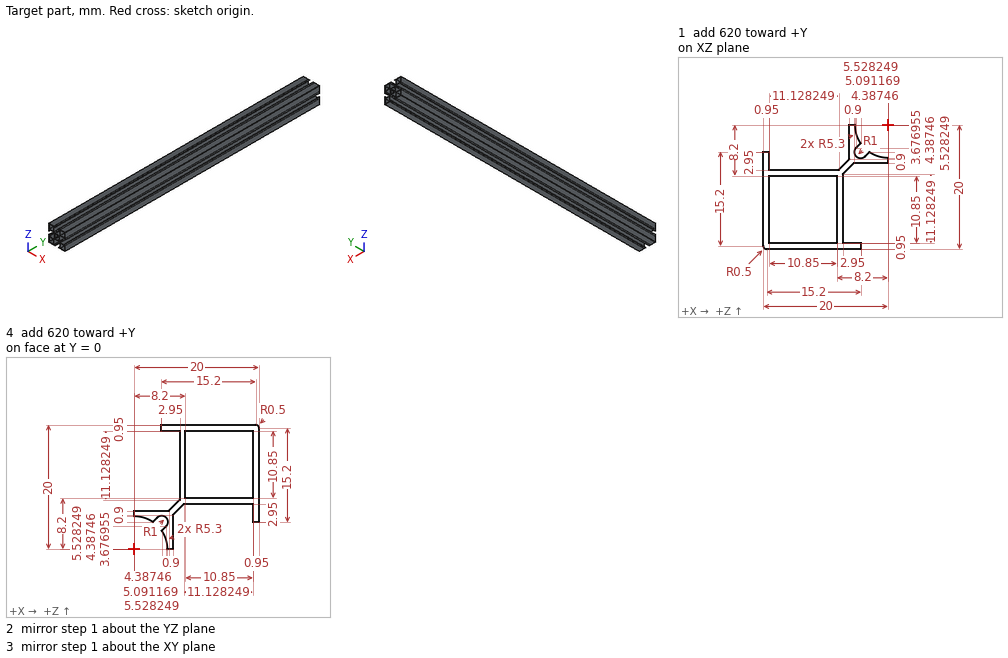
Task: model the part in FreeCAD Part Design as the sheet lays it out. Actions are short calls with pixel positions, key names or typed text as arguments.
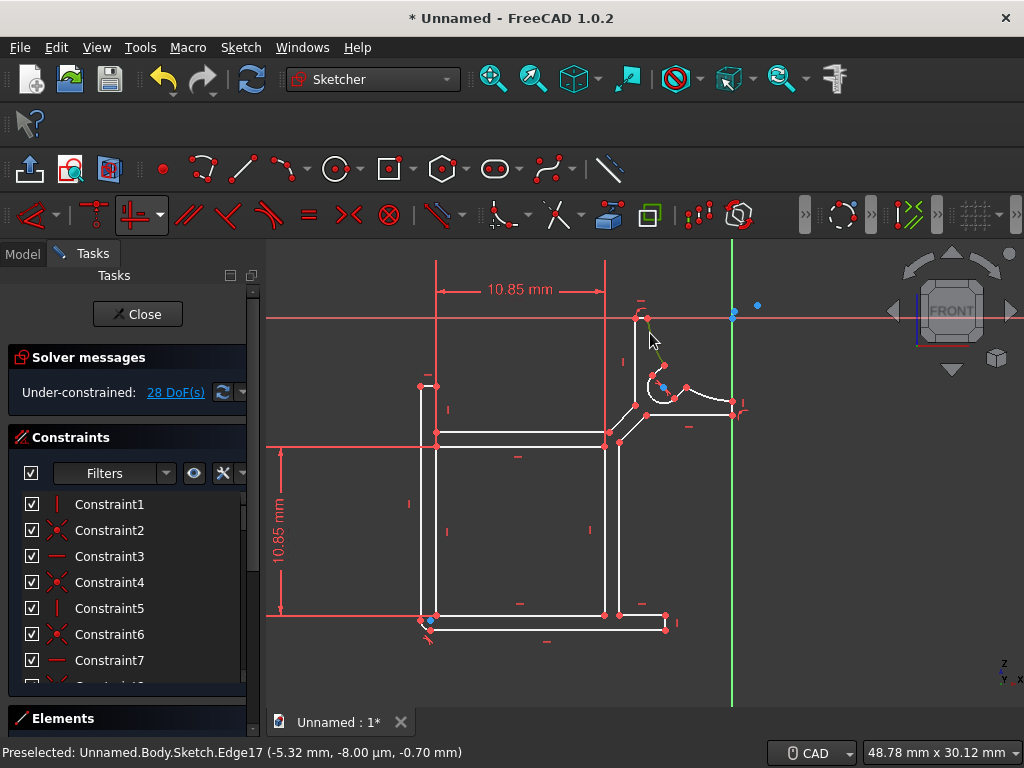
click(699, 394)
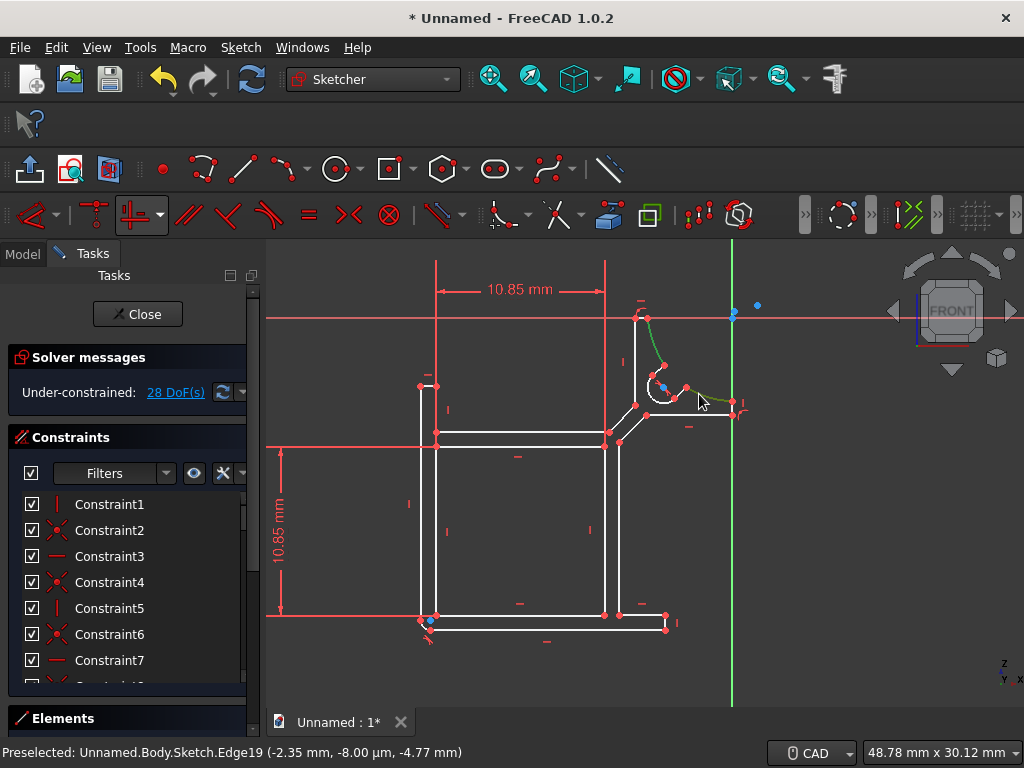
click(94, 216)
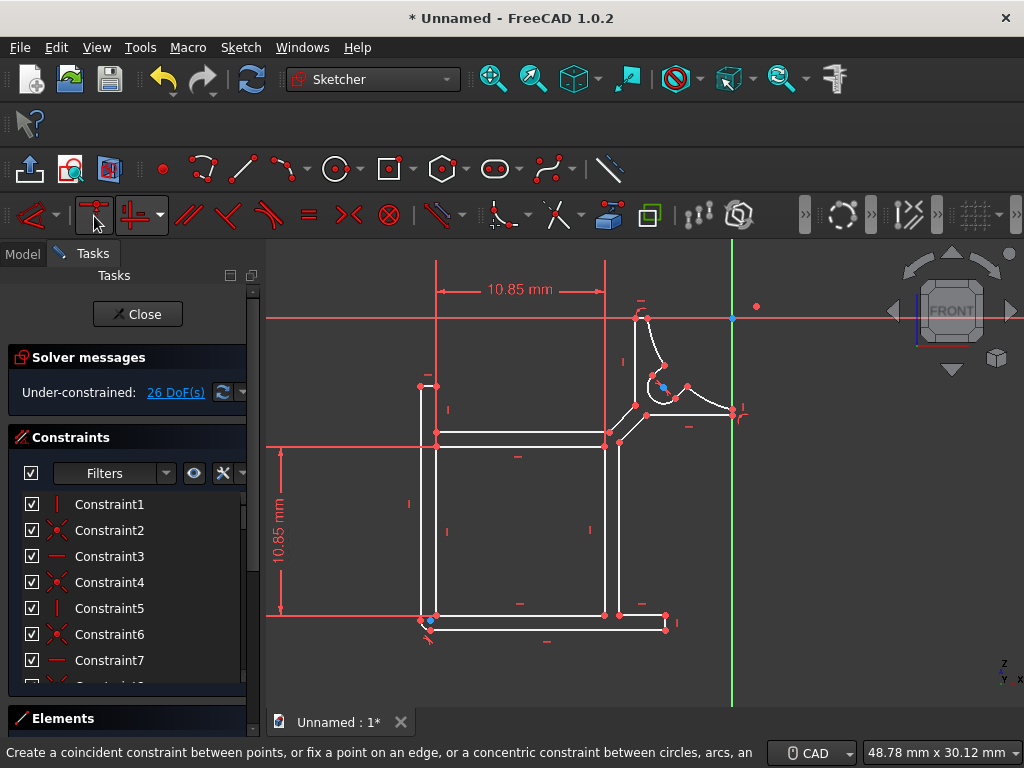
scroll(744, 312, up, 7)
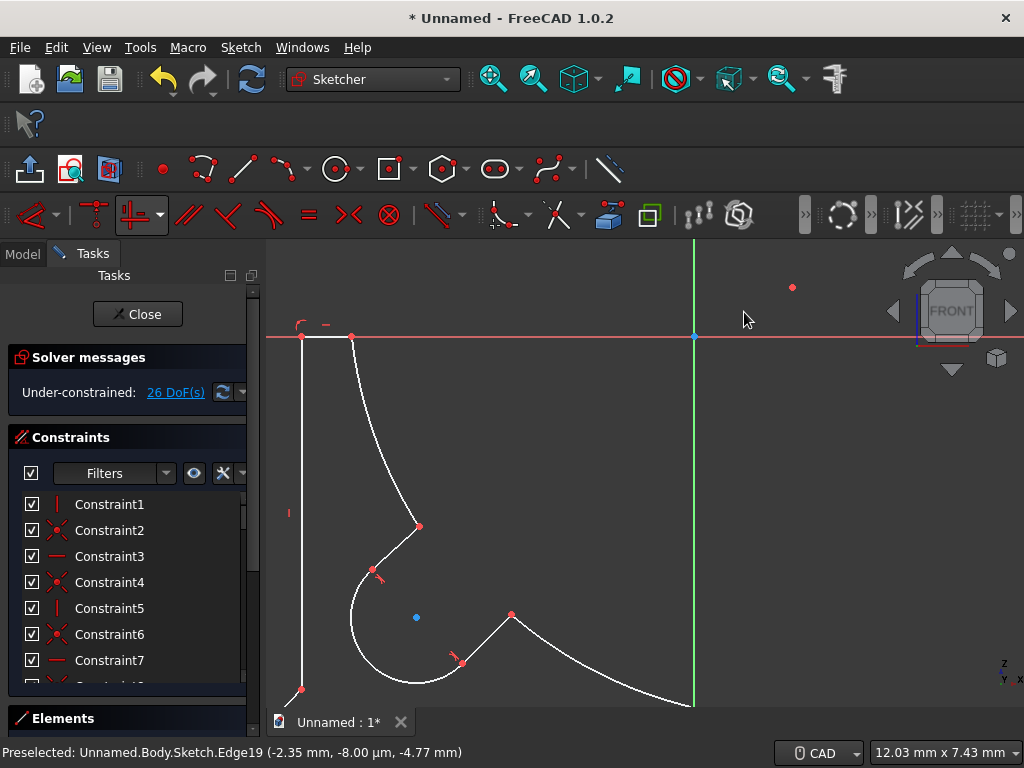
drag(684, 278, 803, 347)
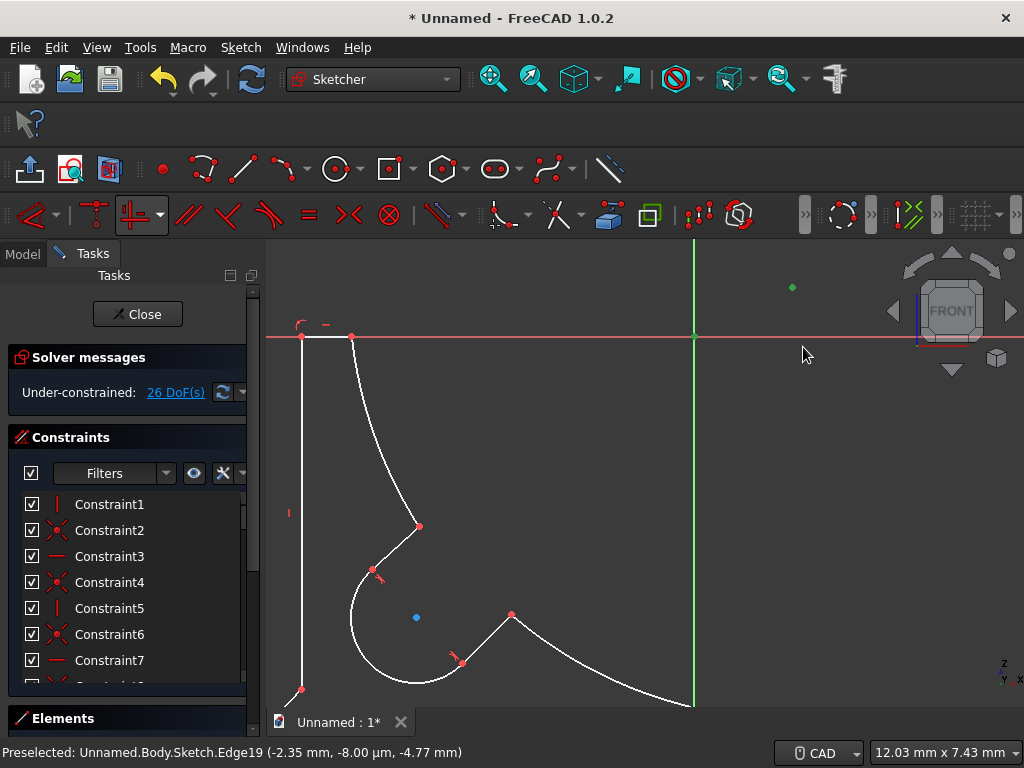
click(94, 216)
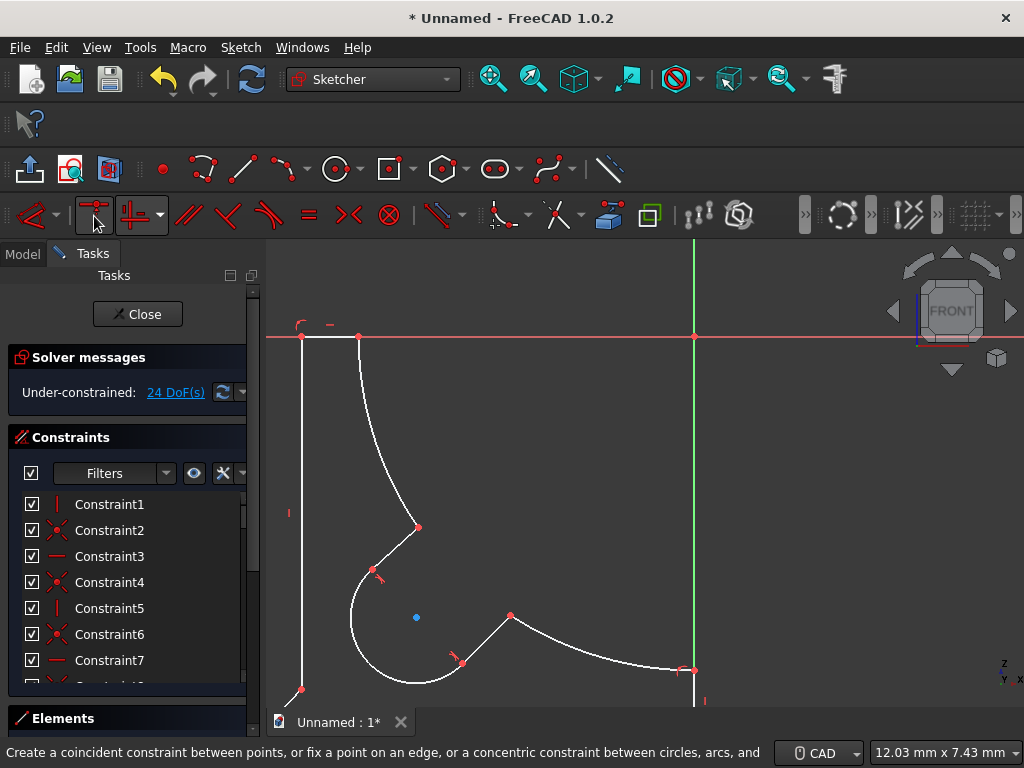
scroll(744, 311, down, 7)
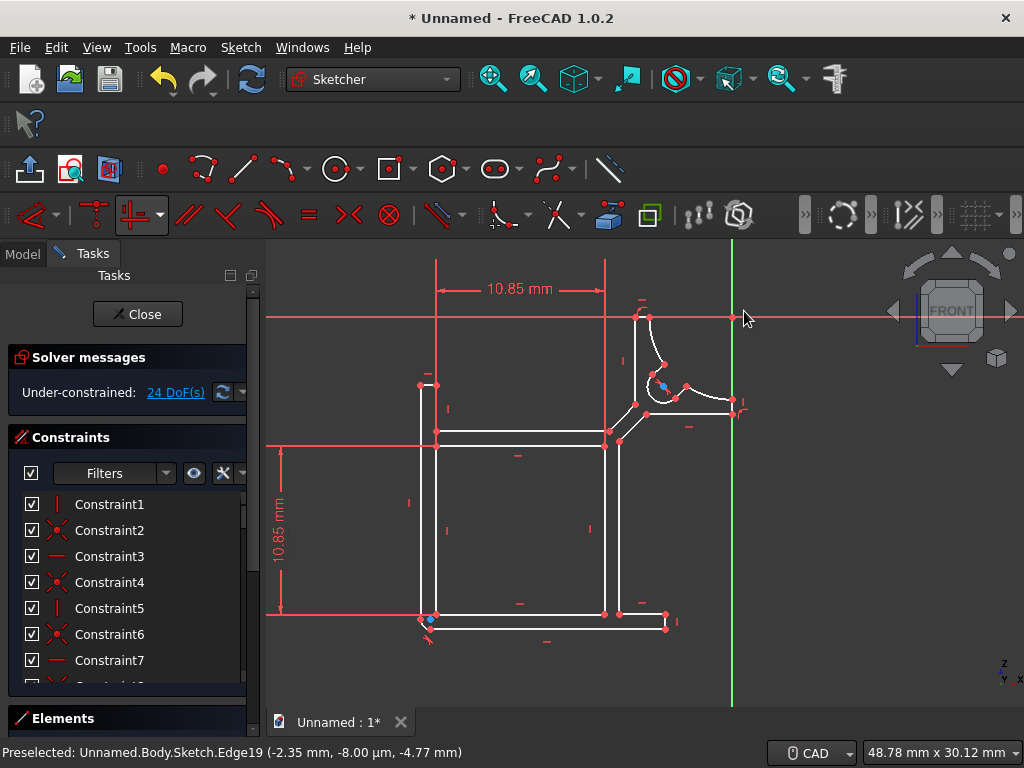
click(651, 332)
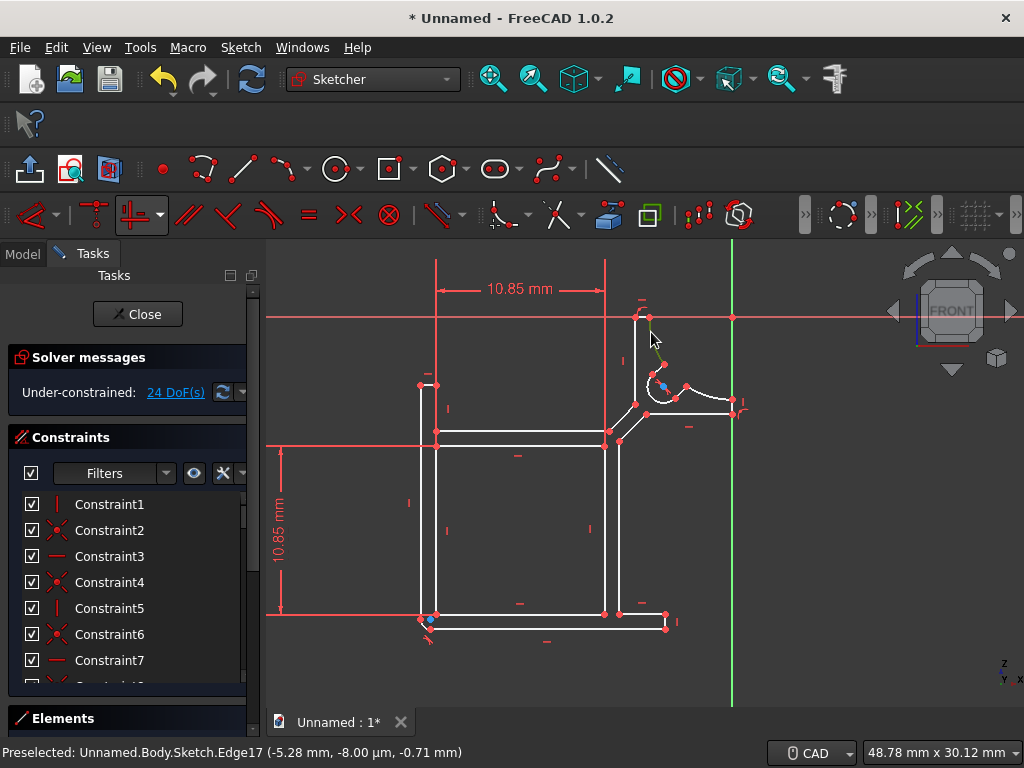
click(700, 393)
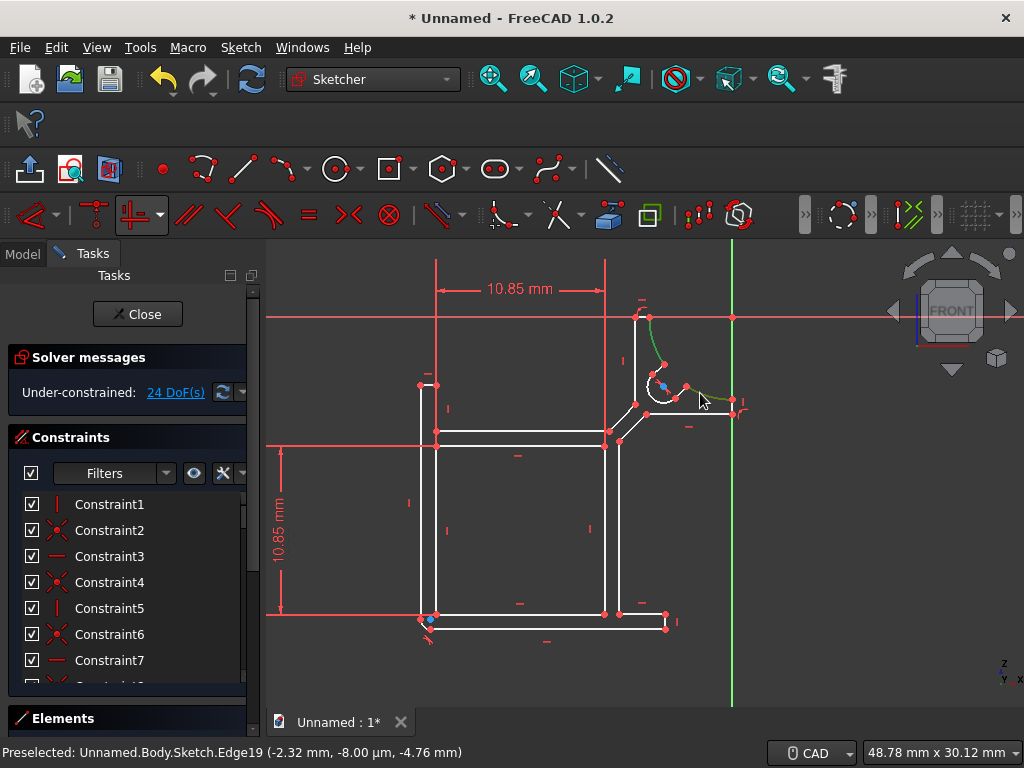
click(310, 216)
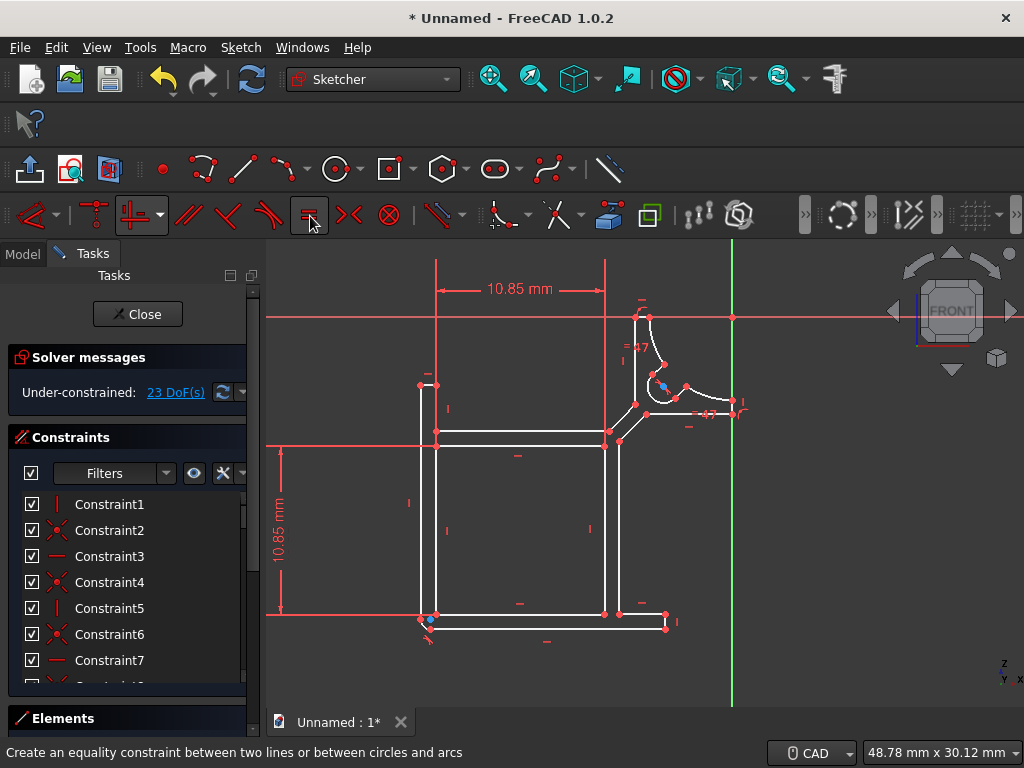
click(651, 332)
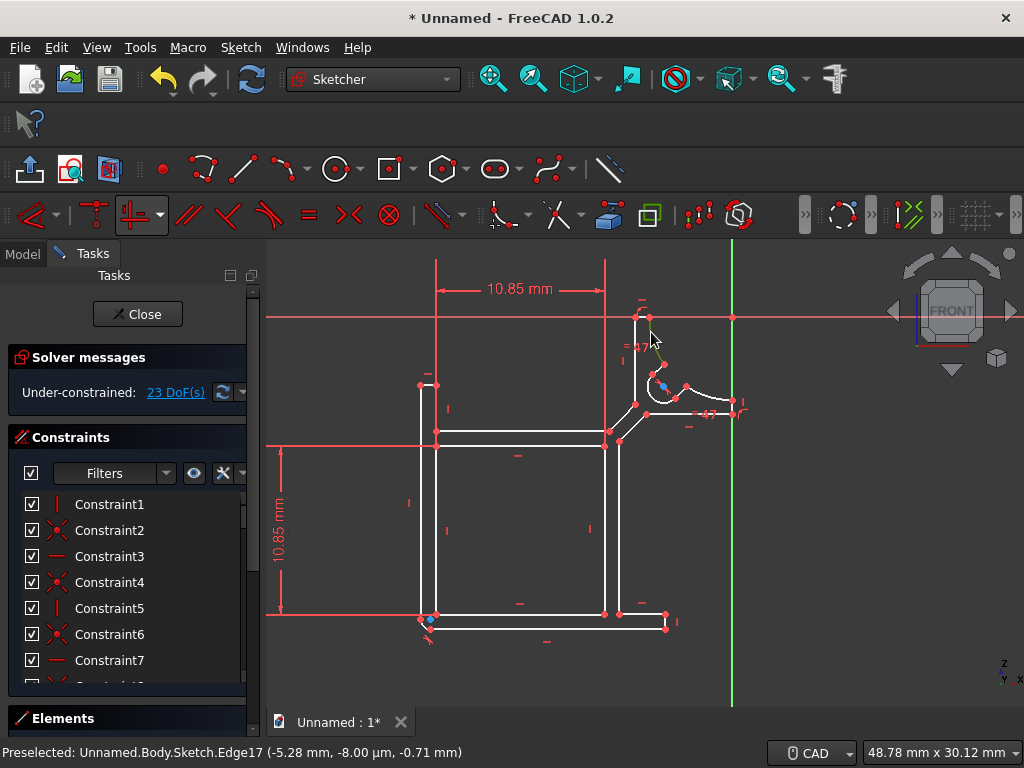
key(k)
key(r)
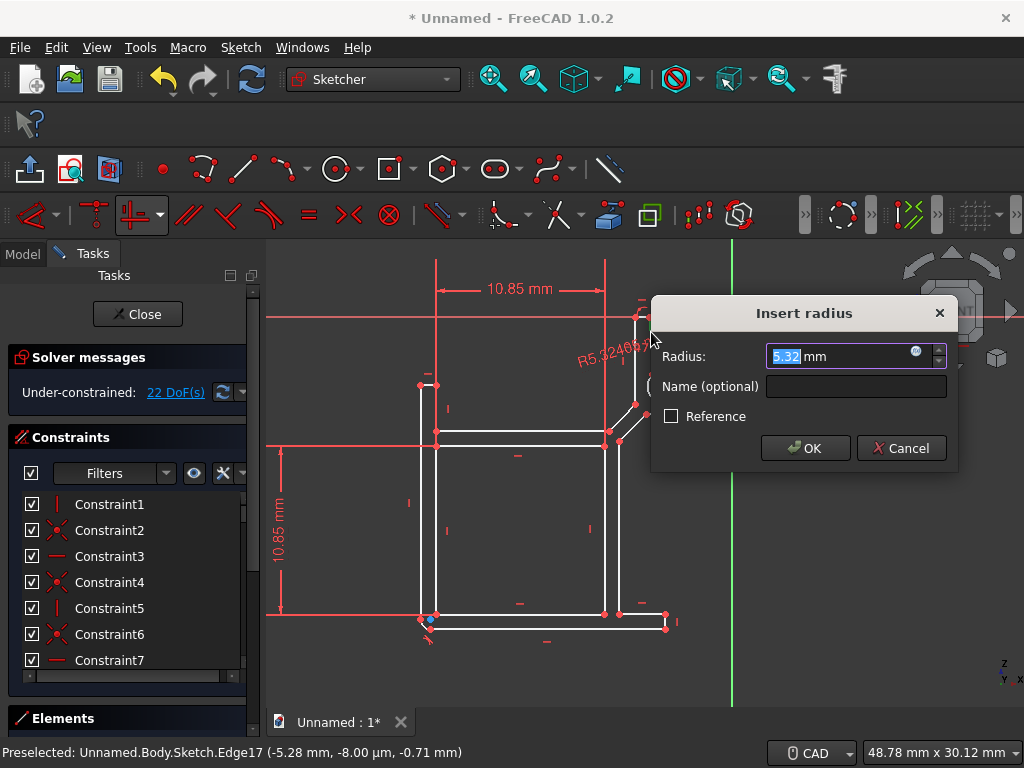
text(5.3)
key(Return)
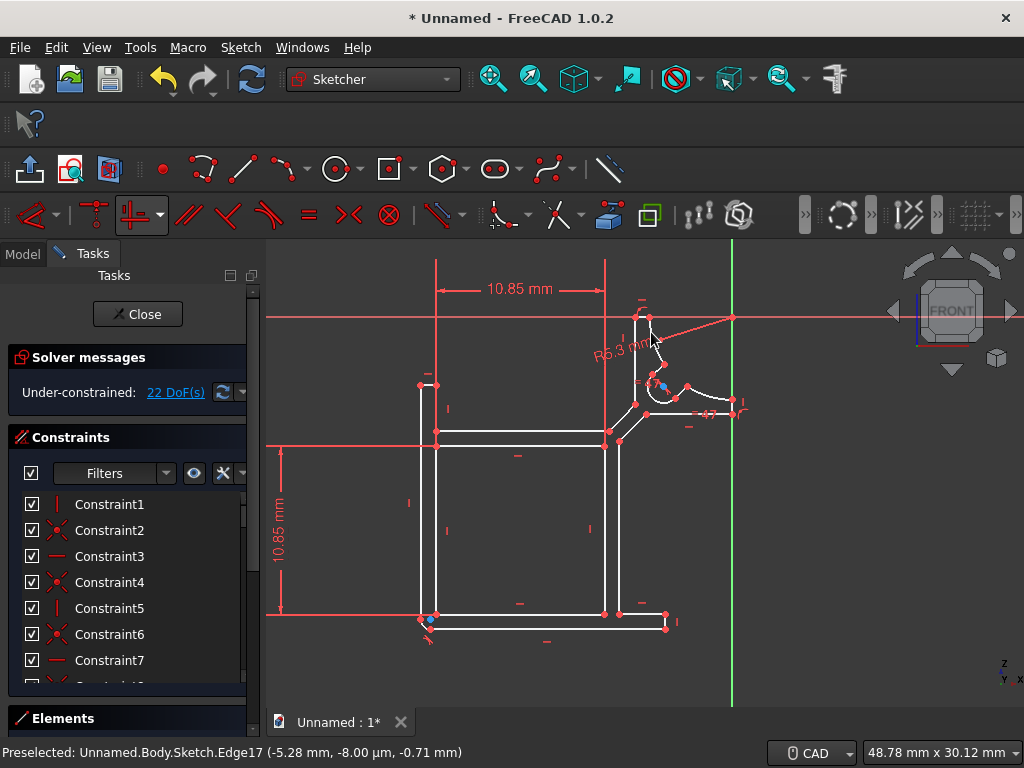
scroll(648, 389, up, 5)